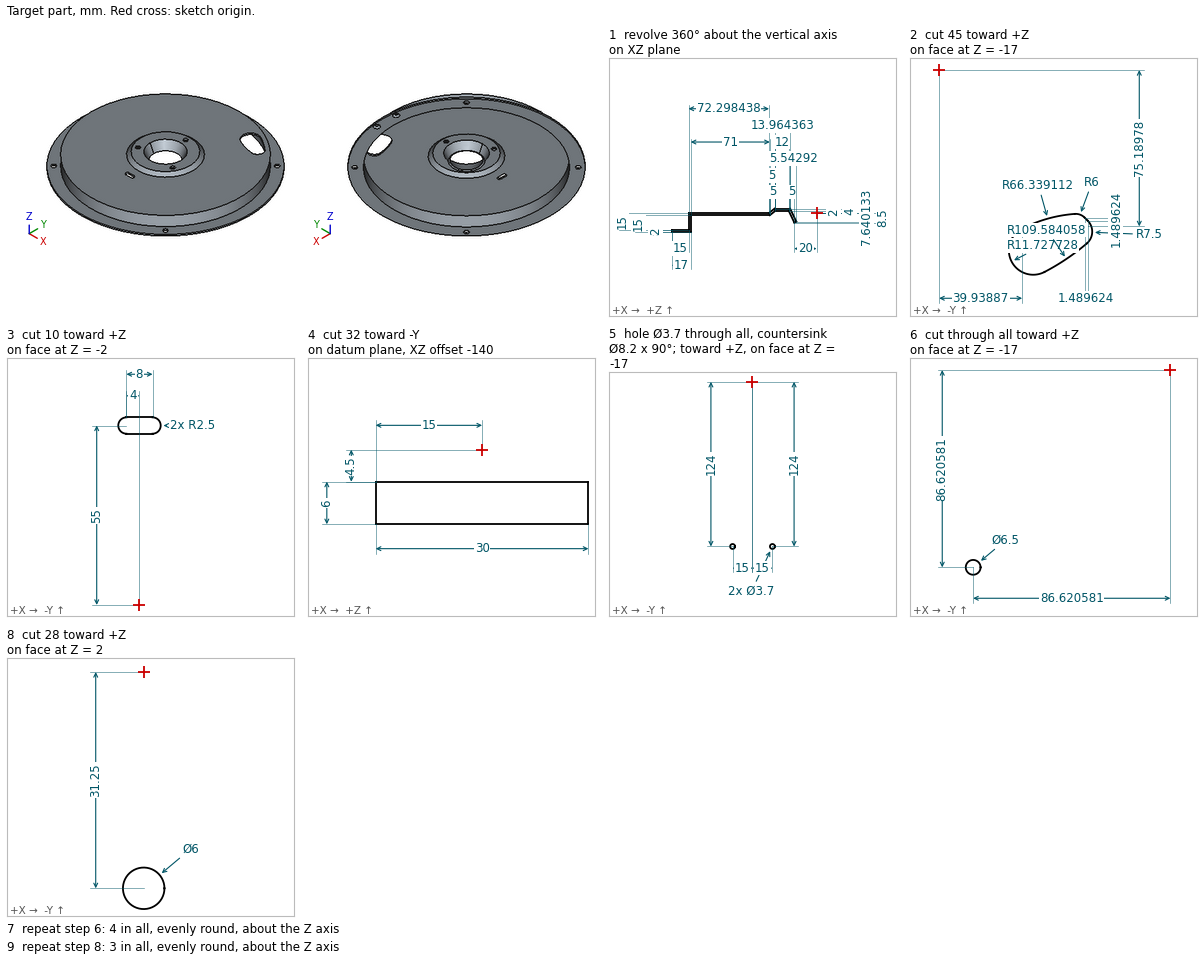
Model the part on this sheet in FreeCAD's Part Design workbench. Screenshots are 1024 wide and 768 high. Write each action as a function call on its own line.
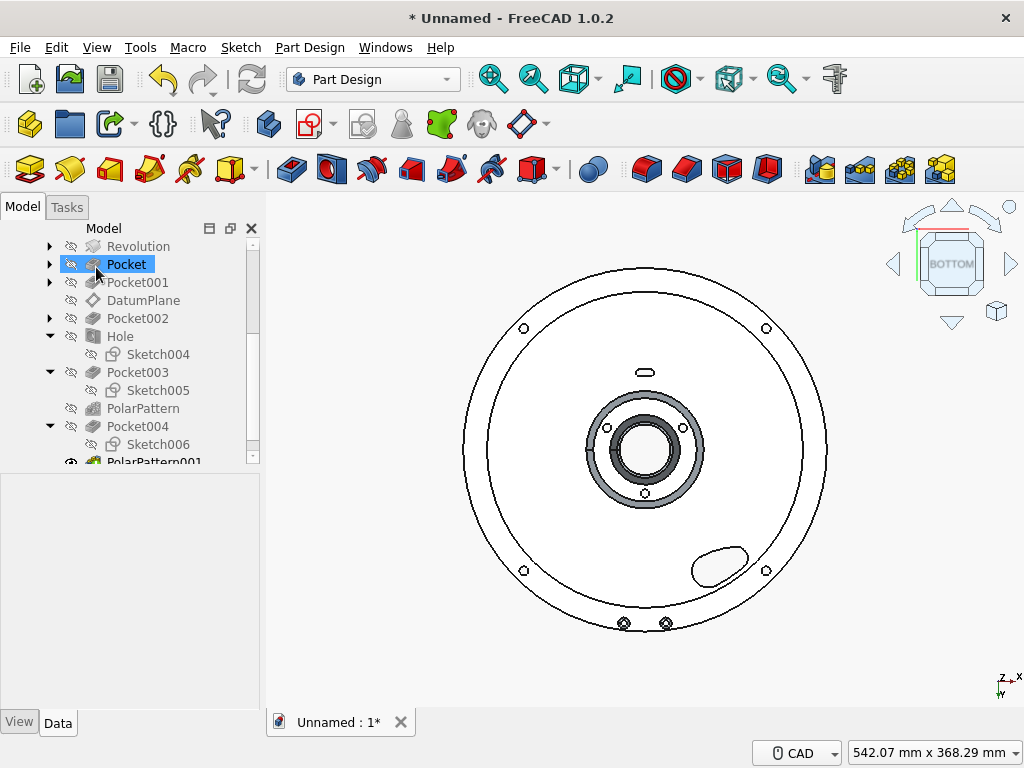
key(0)